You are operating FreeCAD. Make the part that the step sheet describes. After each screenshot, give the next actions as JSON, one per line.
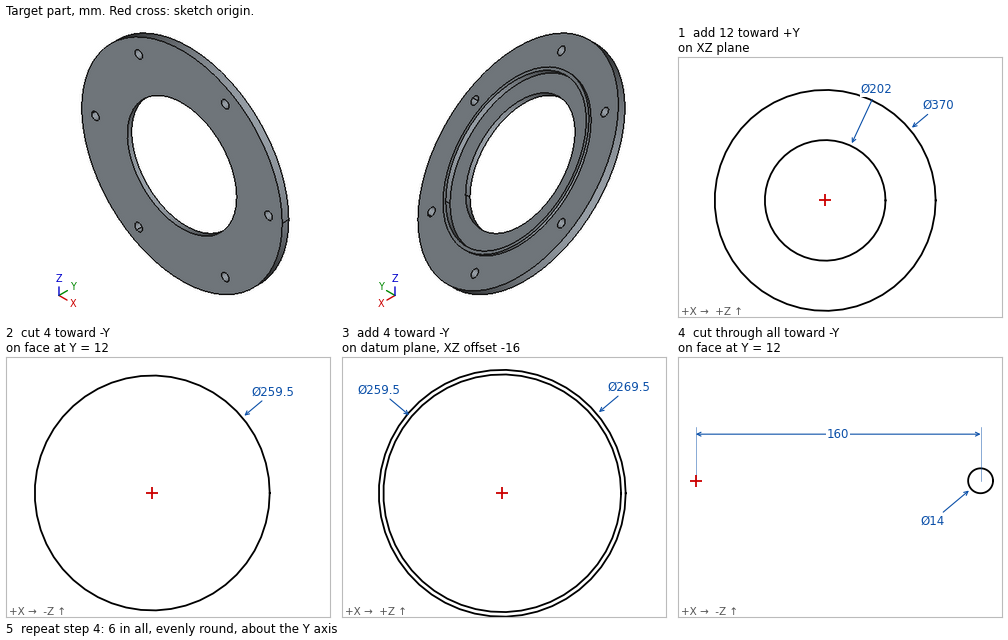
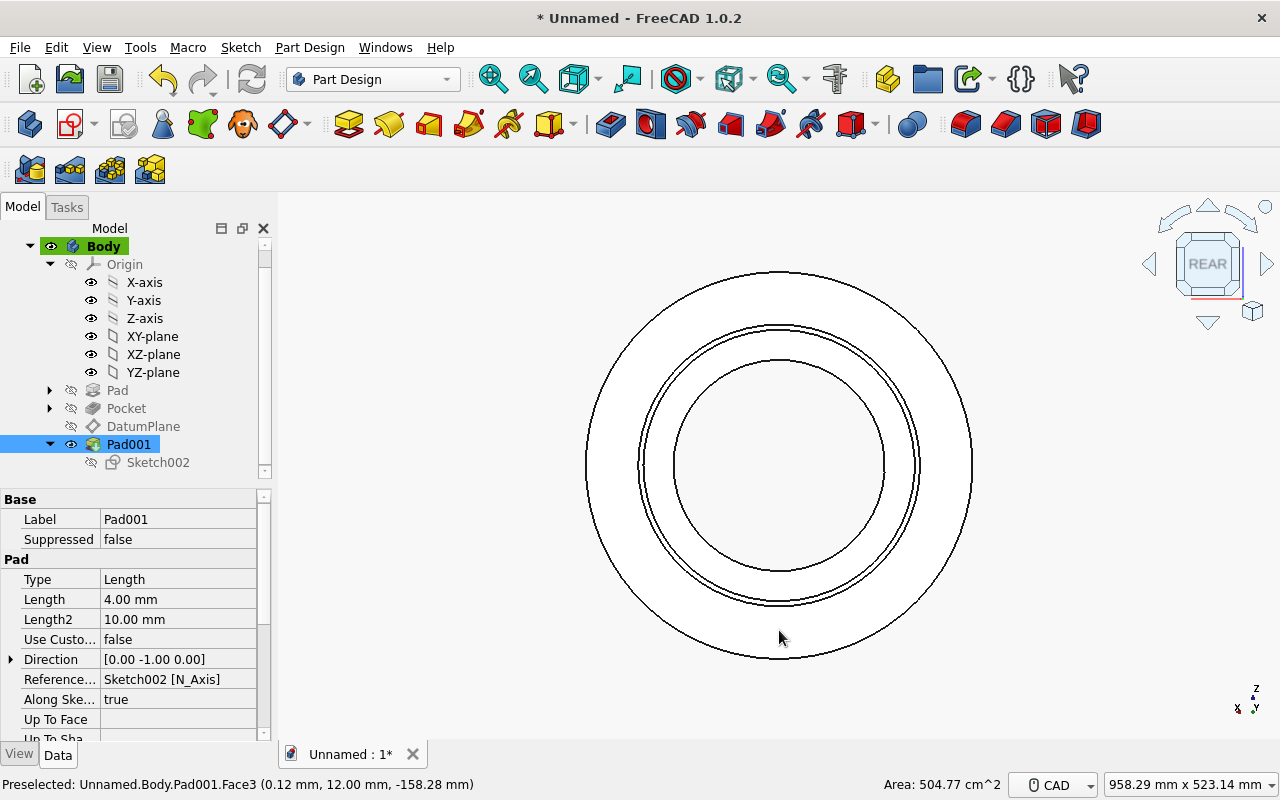
{"action": "left_click", "coordinate": [70, 124]}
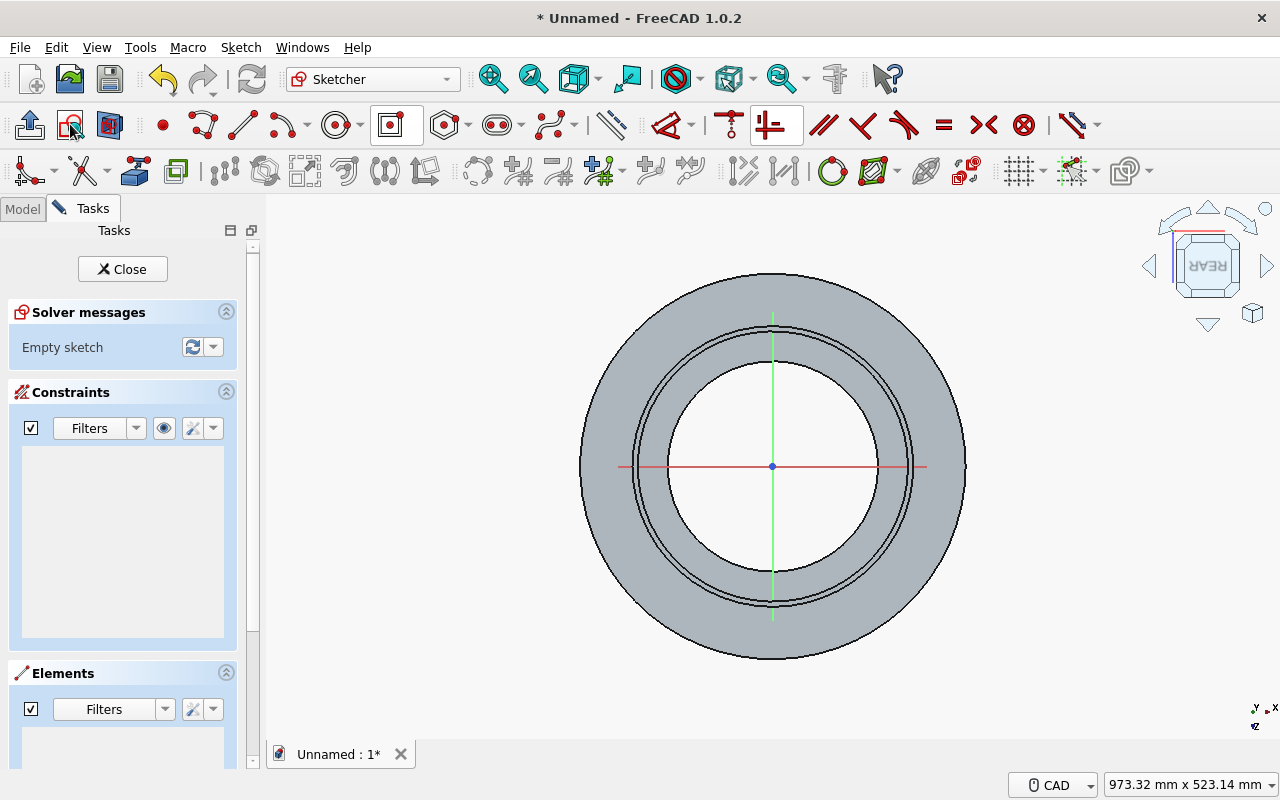
{"action": "left_click", "coordinate": [110, 126]}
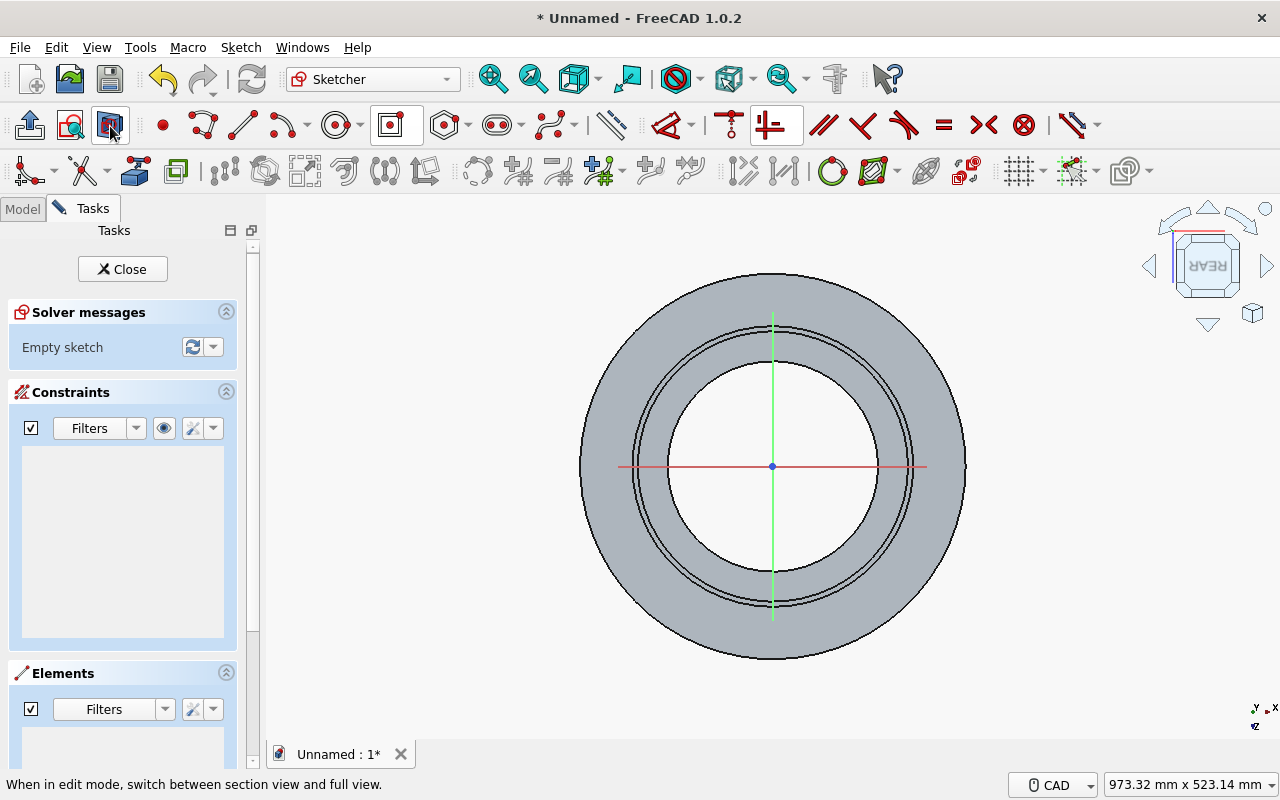
{"action": "scroll", "coordinate": [952, 466], "scroll_direction": "up", "scroll_amount": 15}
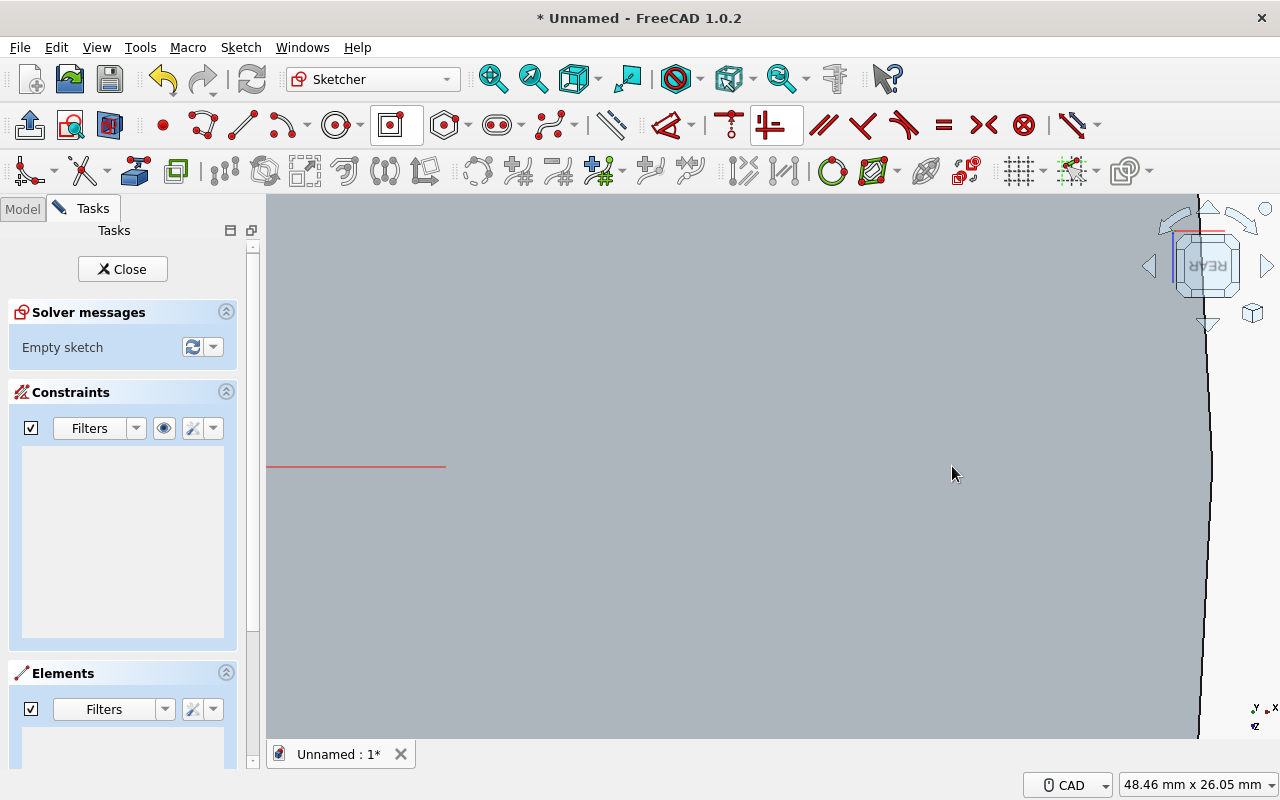
{"action": "left_click", "coordinate": [336, 126]}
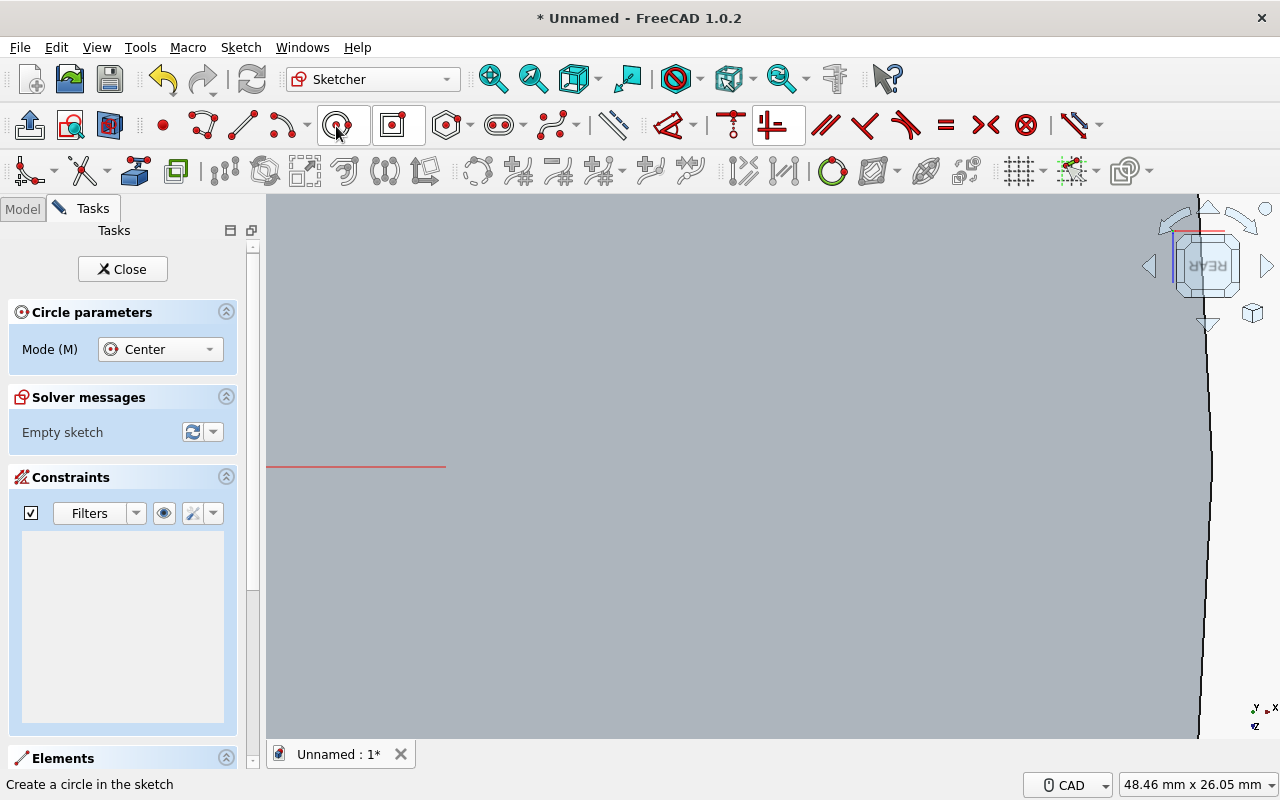
{"action": "left_click", "coordinate": [689, 466]}
{"action": "mouse_move", "coordinate": [793, 363]}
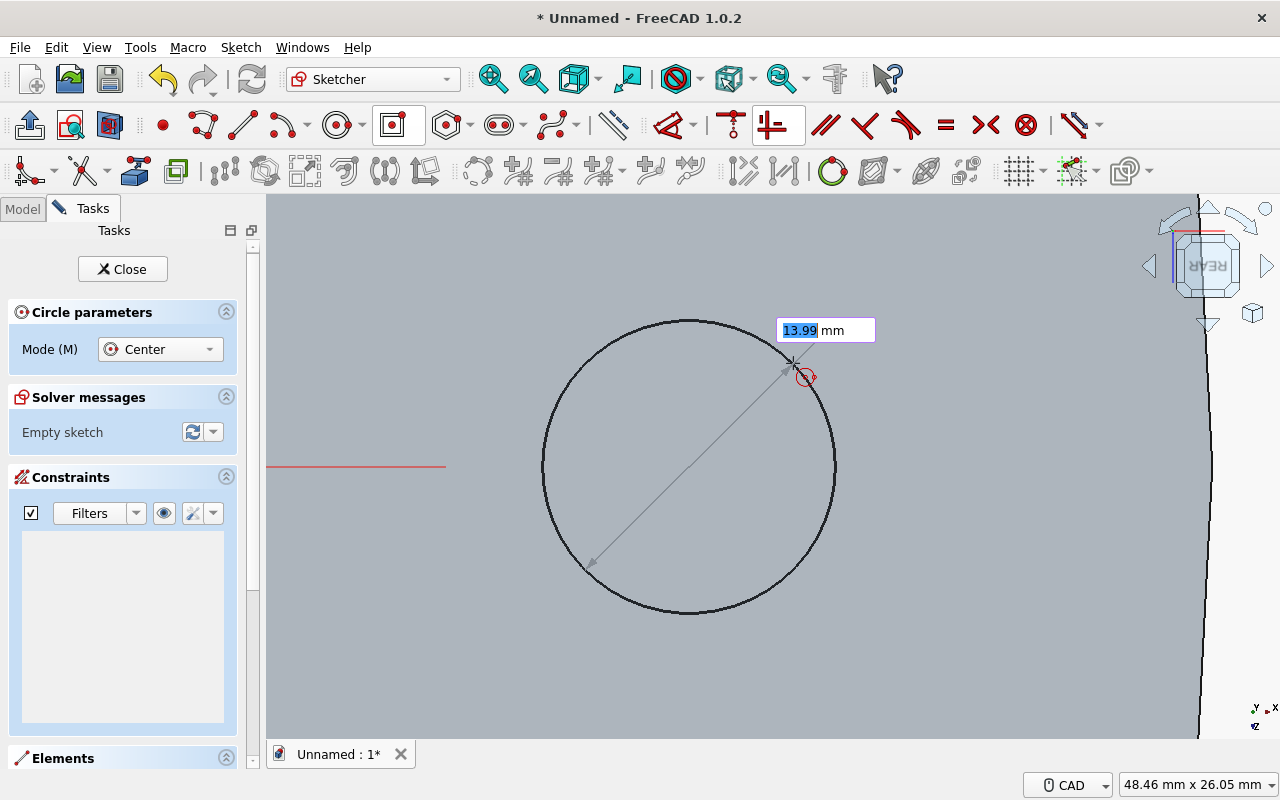
{"action": "type", "text": "14"}
{"action": "key", "text": "Return"}
{"action": "key", "text": "Escape"}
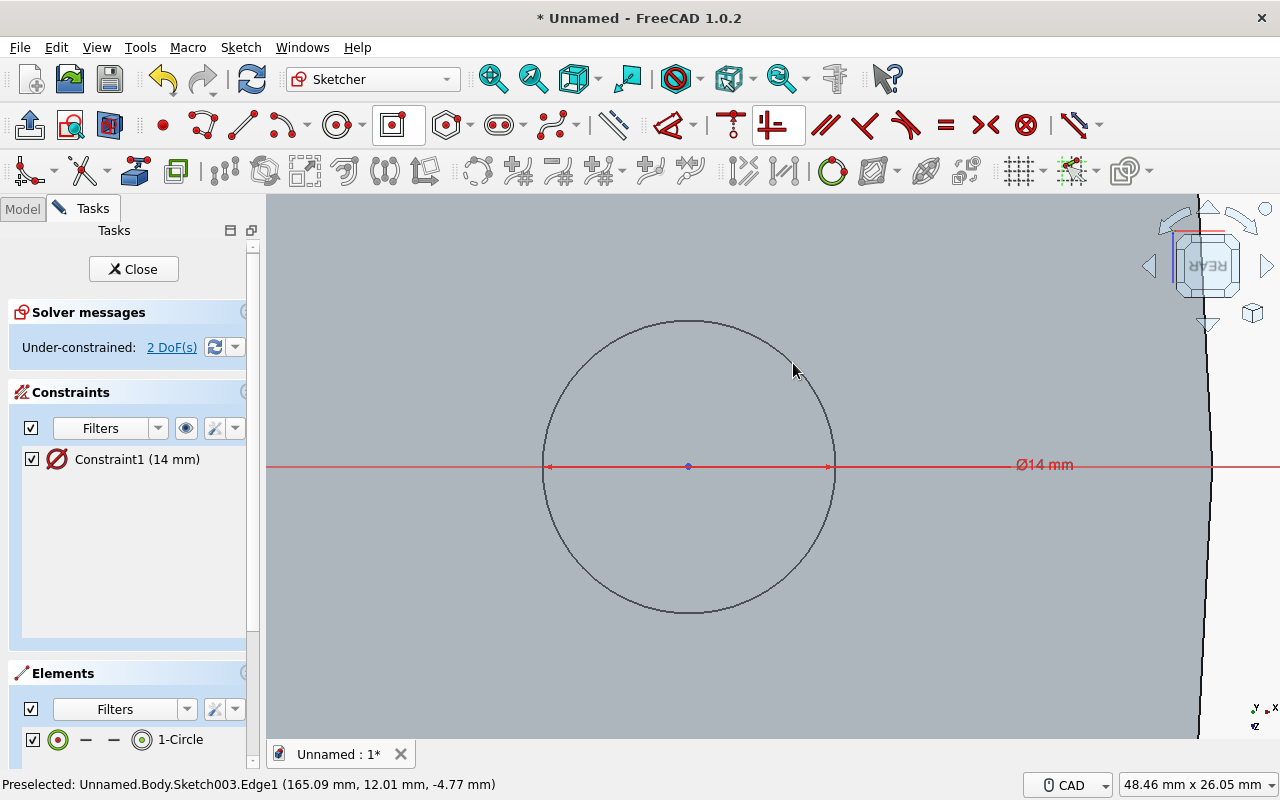
{"action": "left_click", "coordinate": [689, 467]}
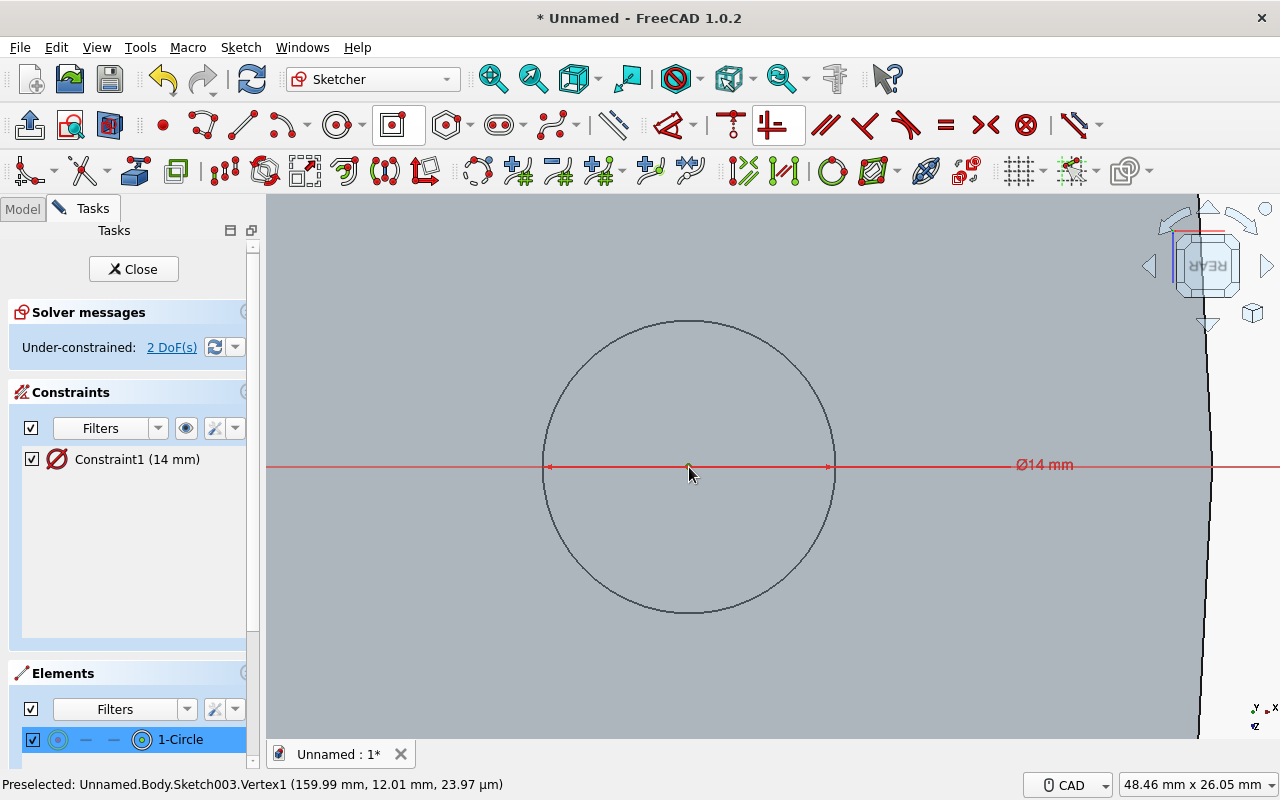
{"action": "left_click", "coordinate": [353, 466]}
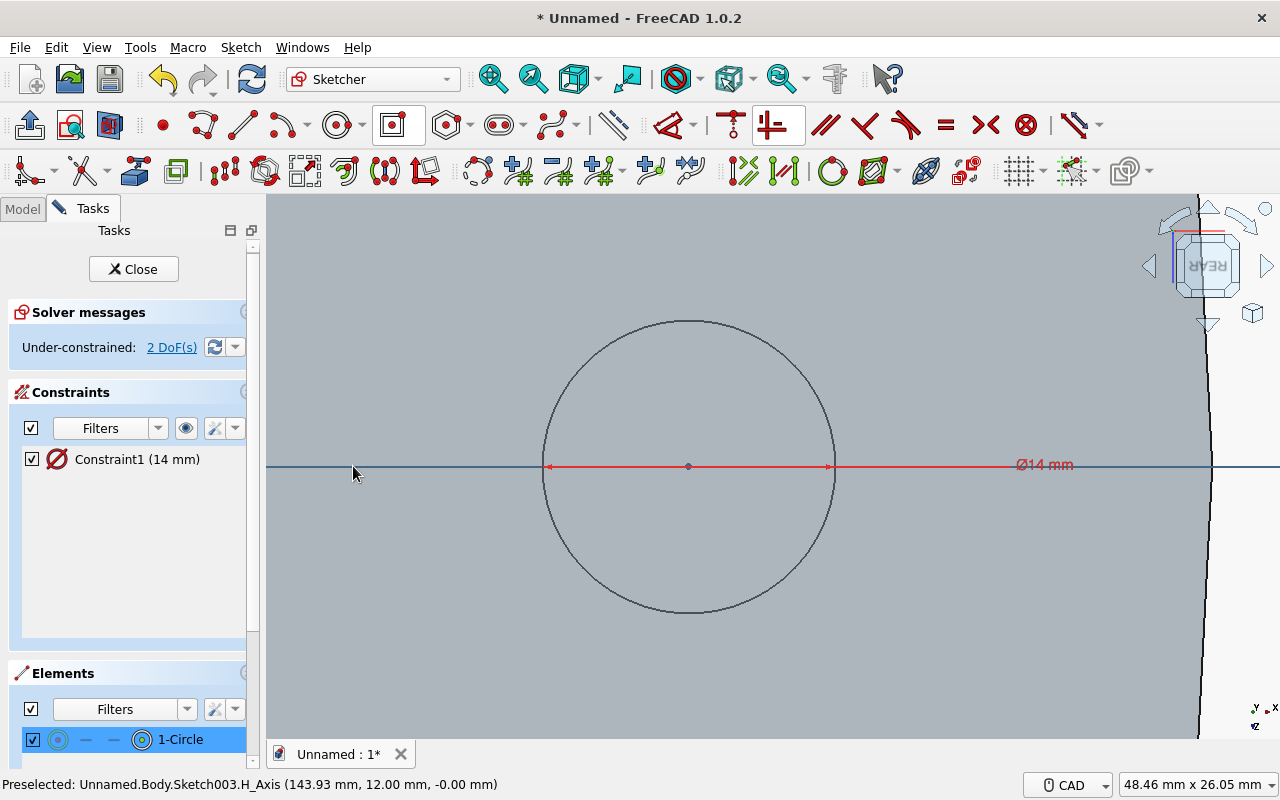
{"action": "left_click", "coordinate": [732, 126]}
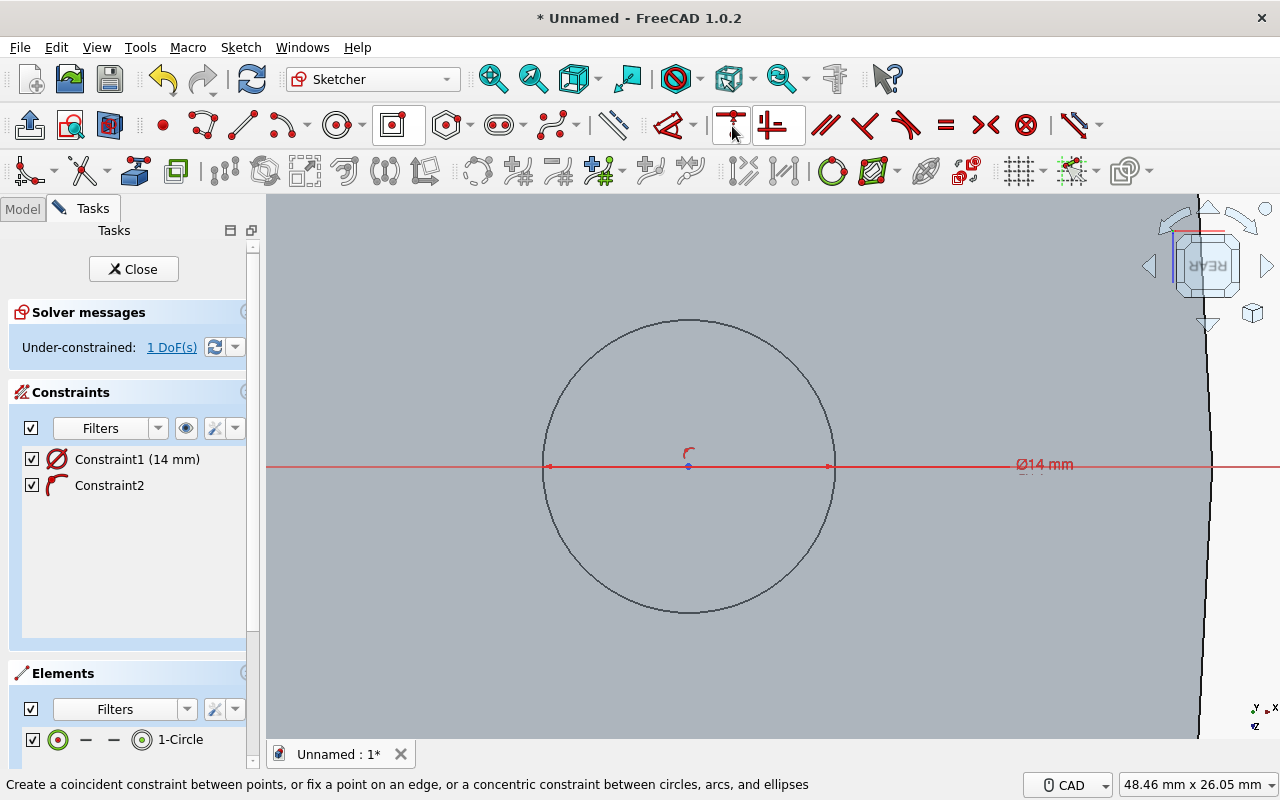
{"action": "left_click", "coordinate": [668, 126]}